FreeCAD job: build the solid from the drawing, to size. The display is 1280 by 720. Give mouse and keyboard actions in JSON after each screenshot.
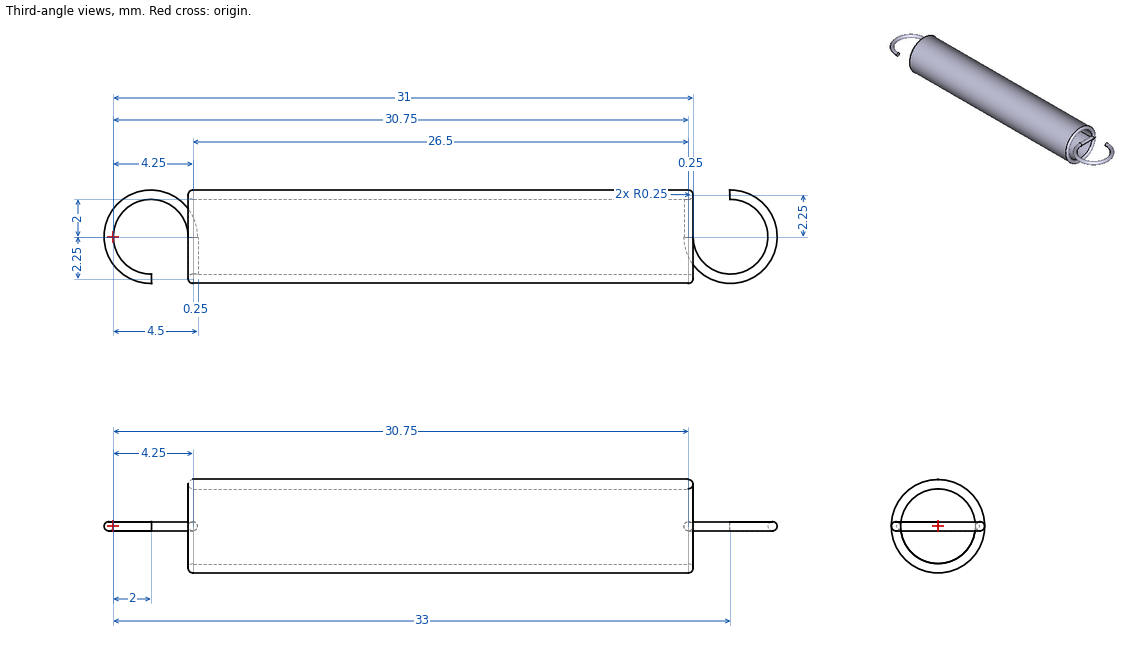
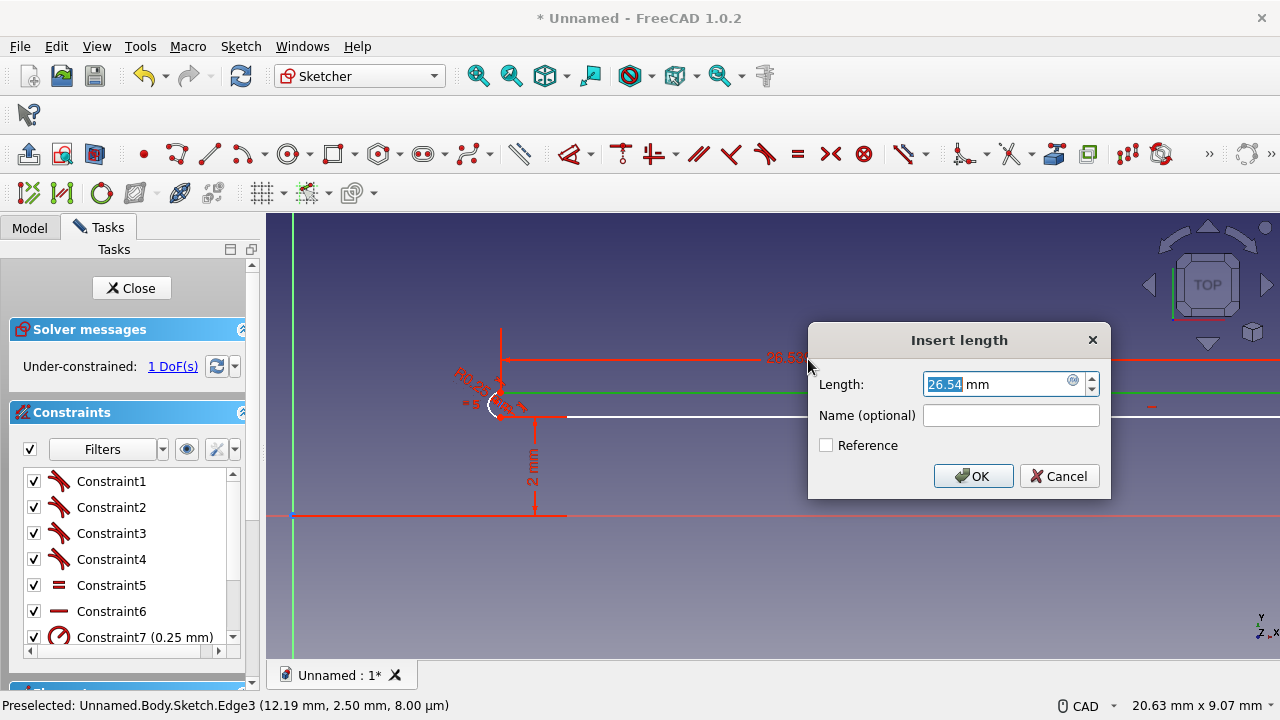
{"action": "type", "text": "26.5"}
{"action": "key", "text": "Return"}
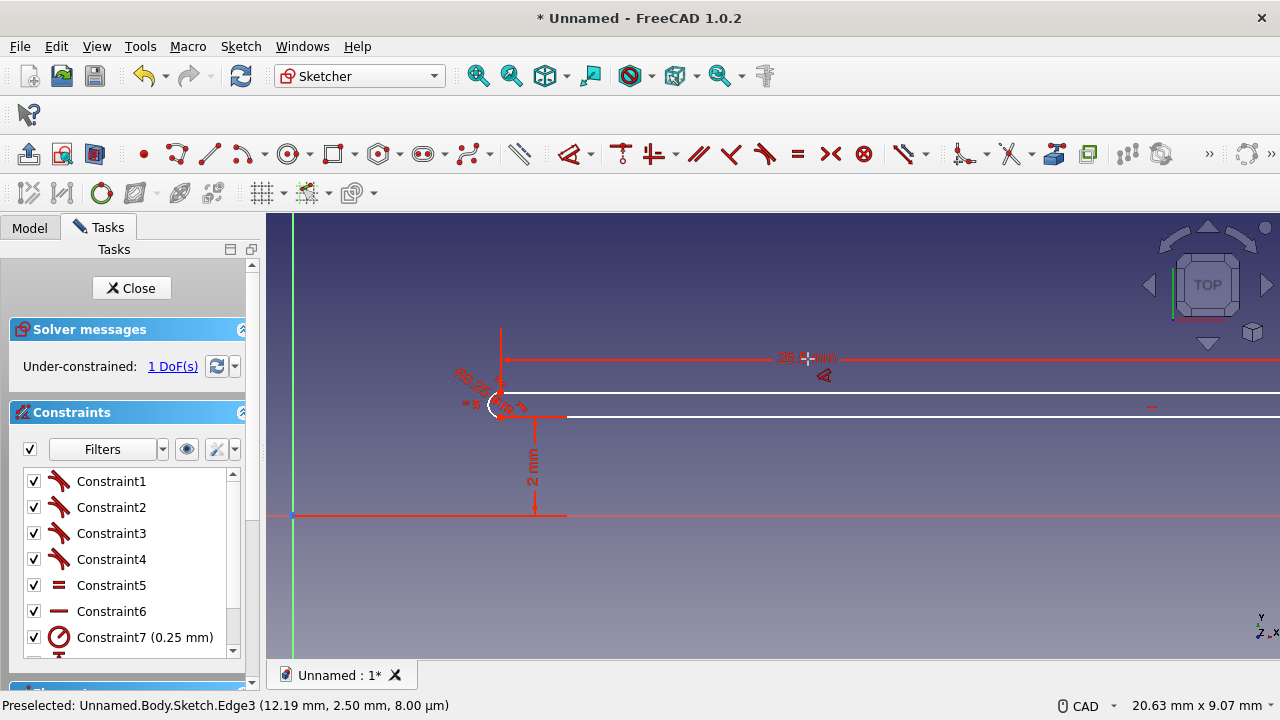
{"action": "left_click", "coordinate": [501, 393]}
{"action": "left_click", "coordinate": [397, 550]}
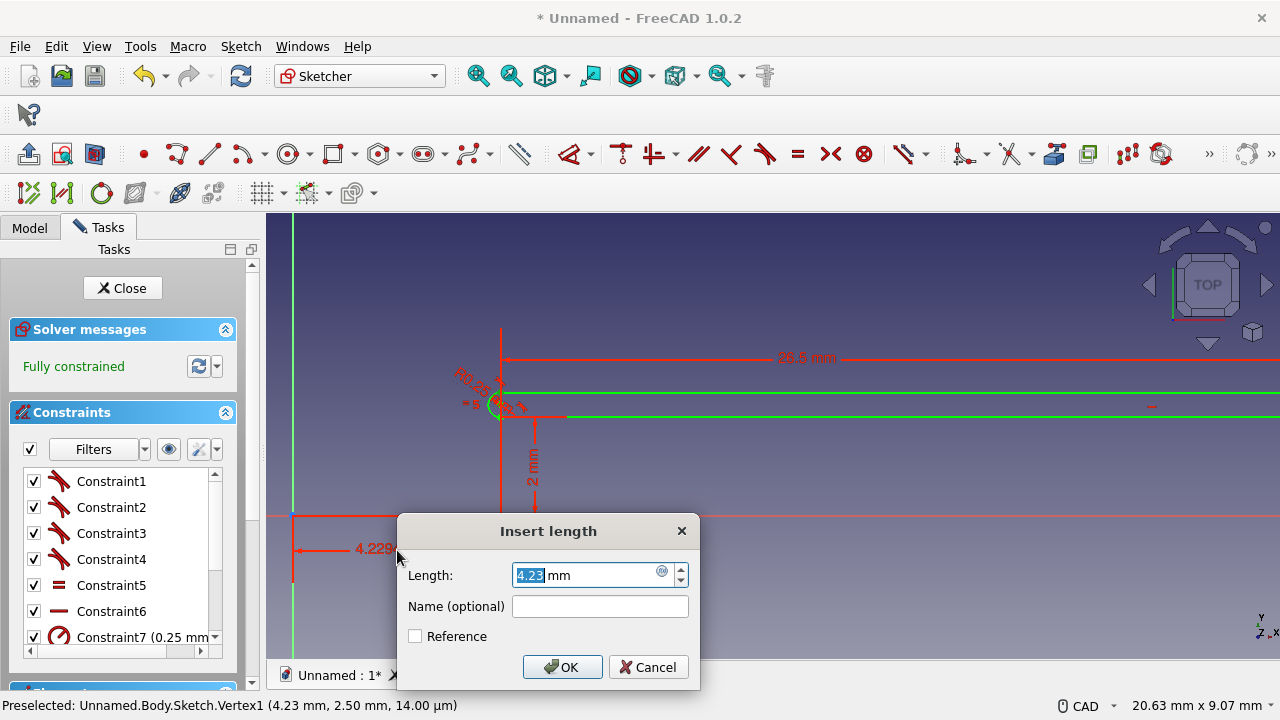
{"action": "type", "text": "4.25"}
{"action": "key", "text": "Return"}
{"action": "key", "text": "Escape"}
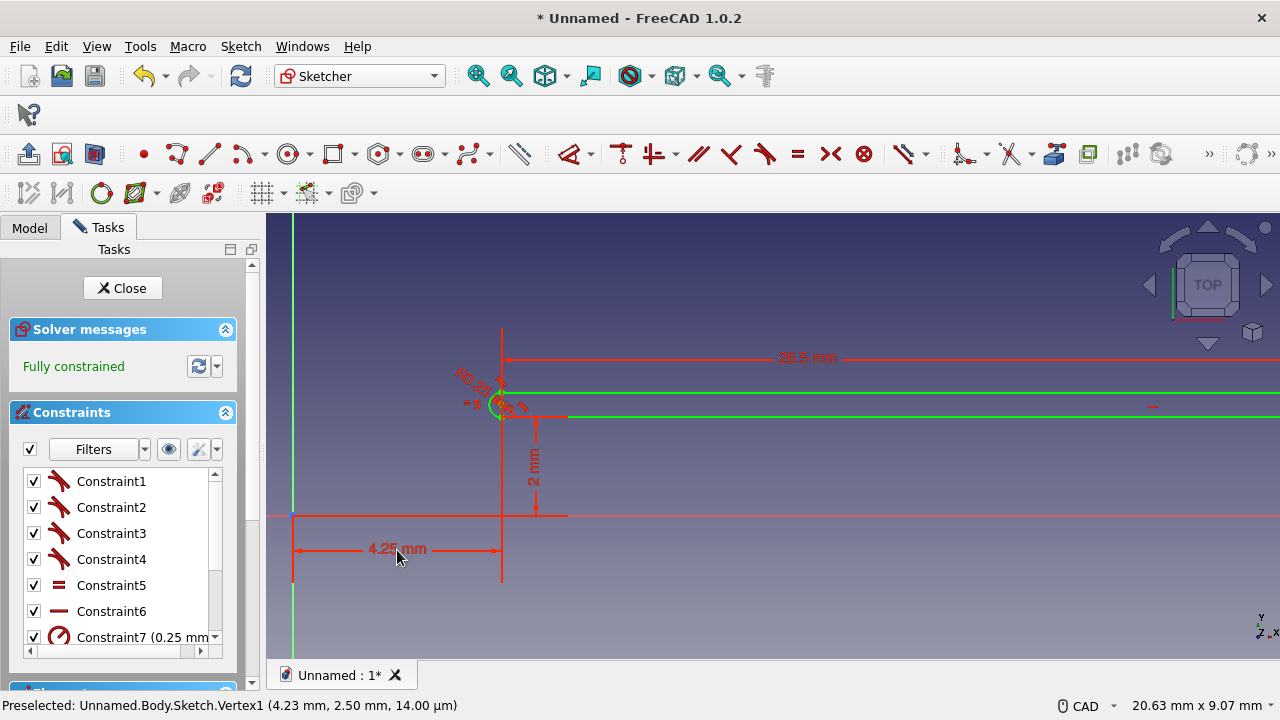
{"action": "left_click", "coordinate": [123, 288]}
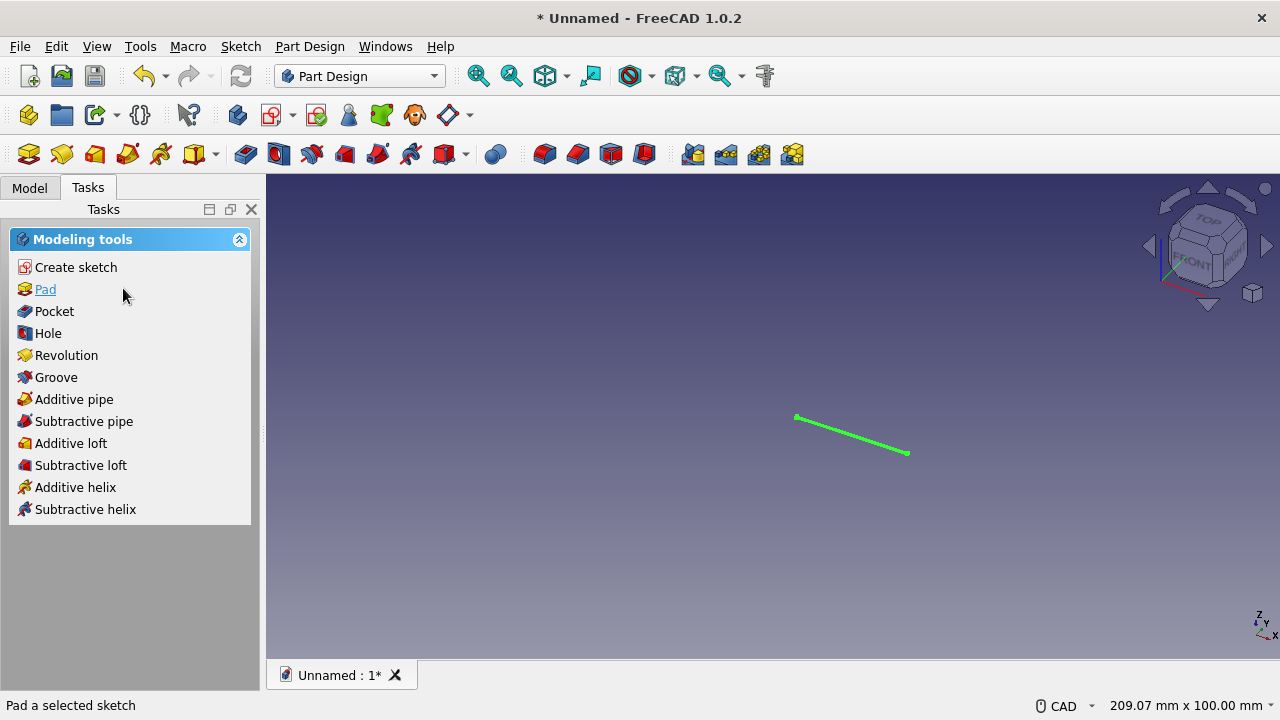
{"action": "left_click", "coordinate": [62, 154]}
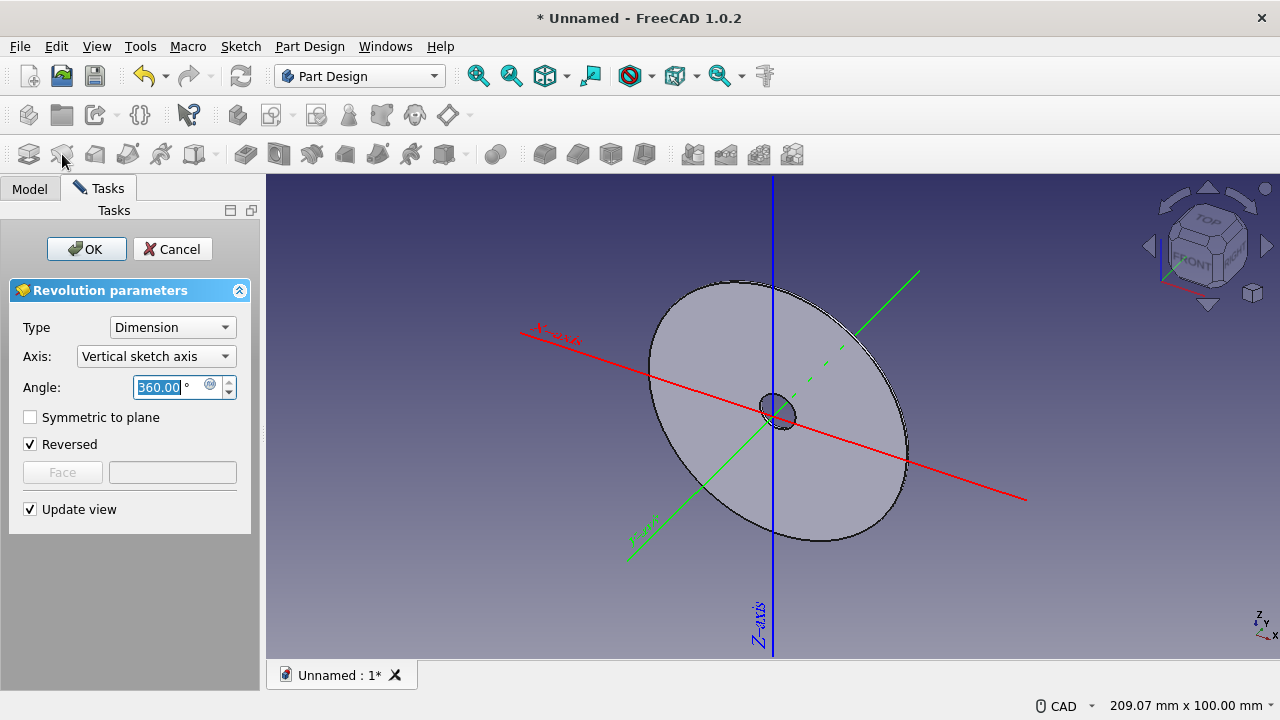
{"action": "left_click", "coordinate": [157, 356]}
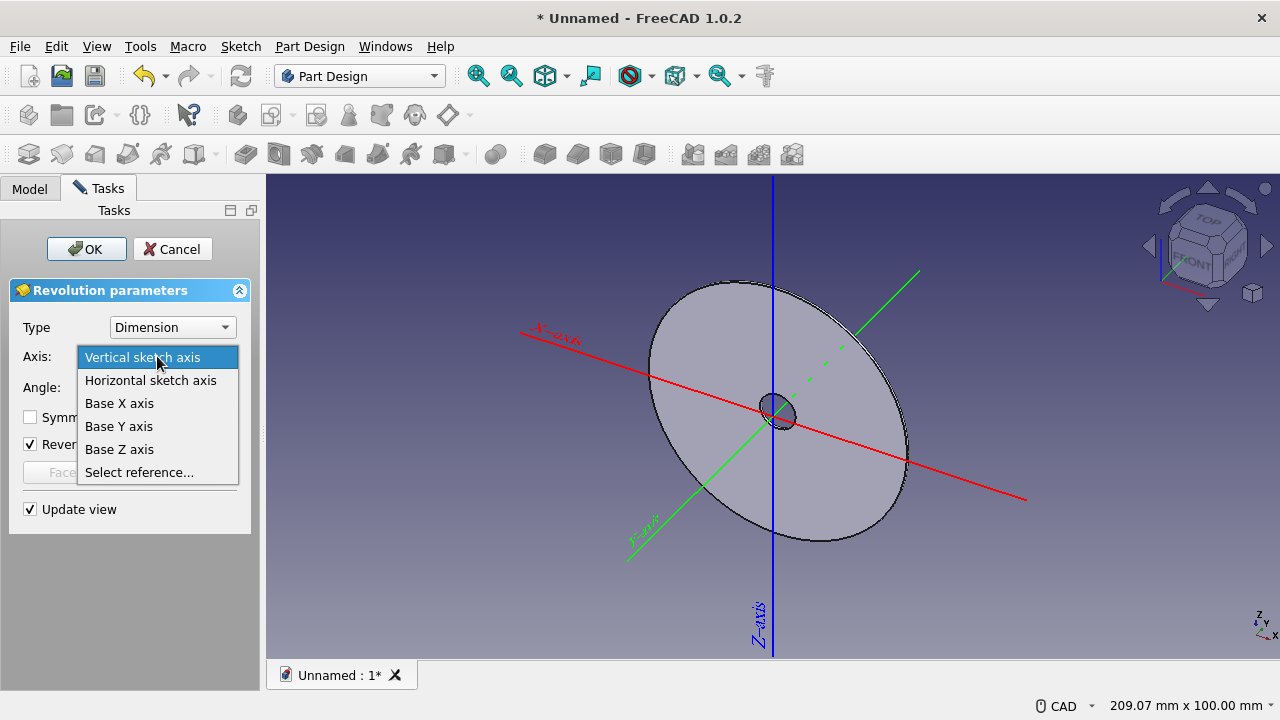
{"action": "left_click", "coordinate": [156, 380]}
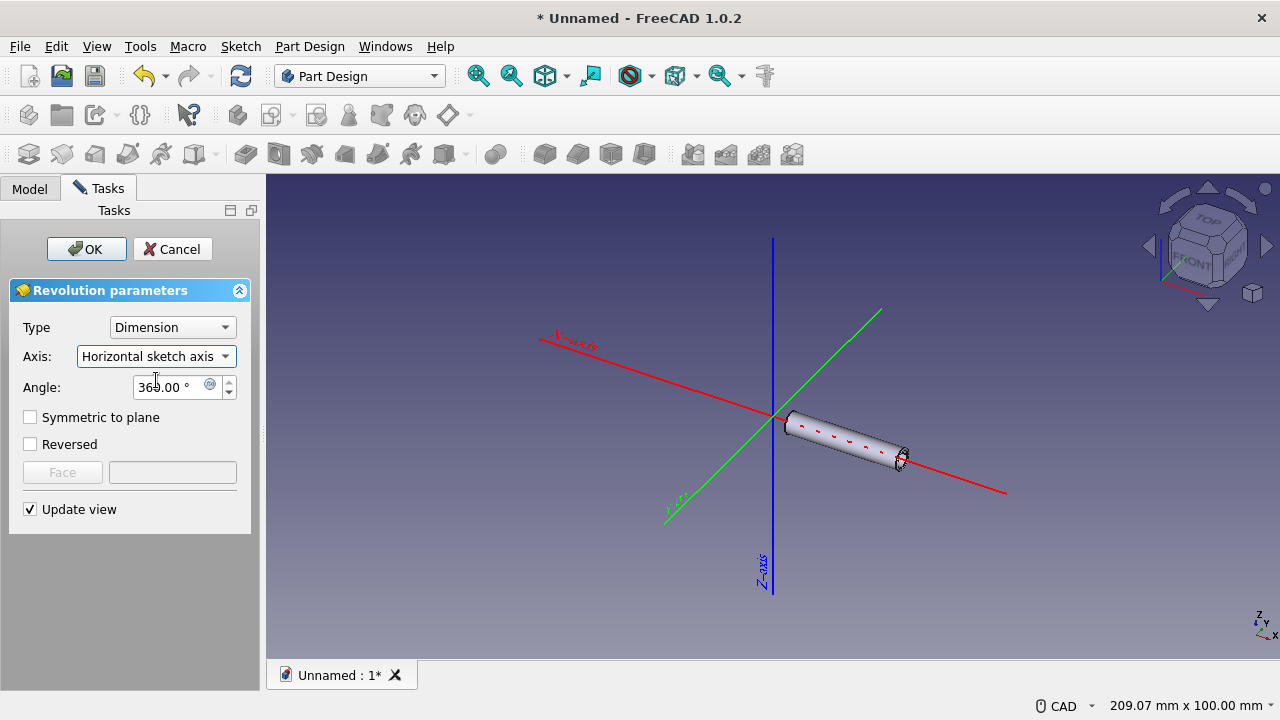
{"action": "left_click", "coordinate": [87, 249]}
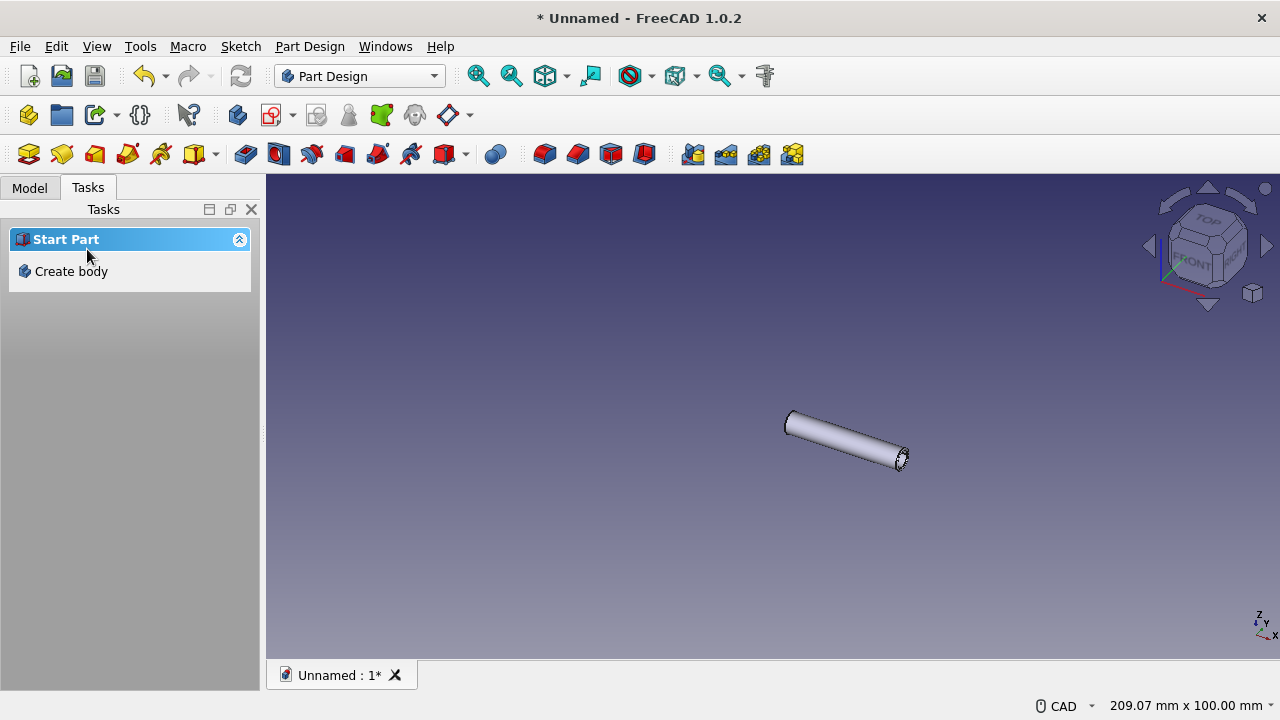
{"action": "key", "text": "v f"}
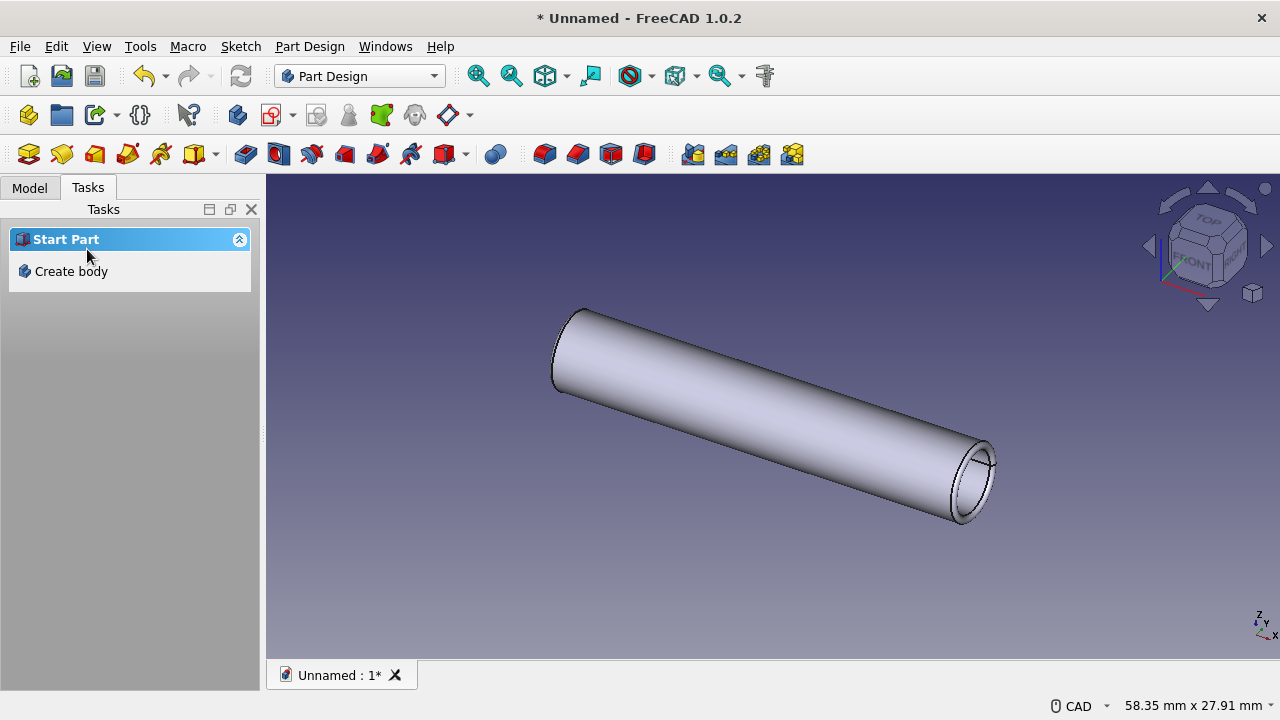
{"action": "left_click", "coordinate": [270, 116]}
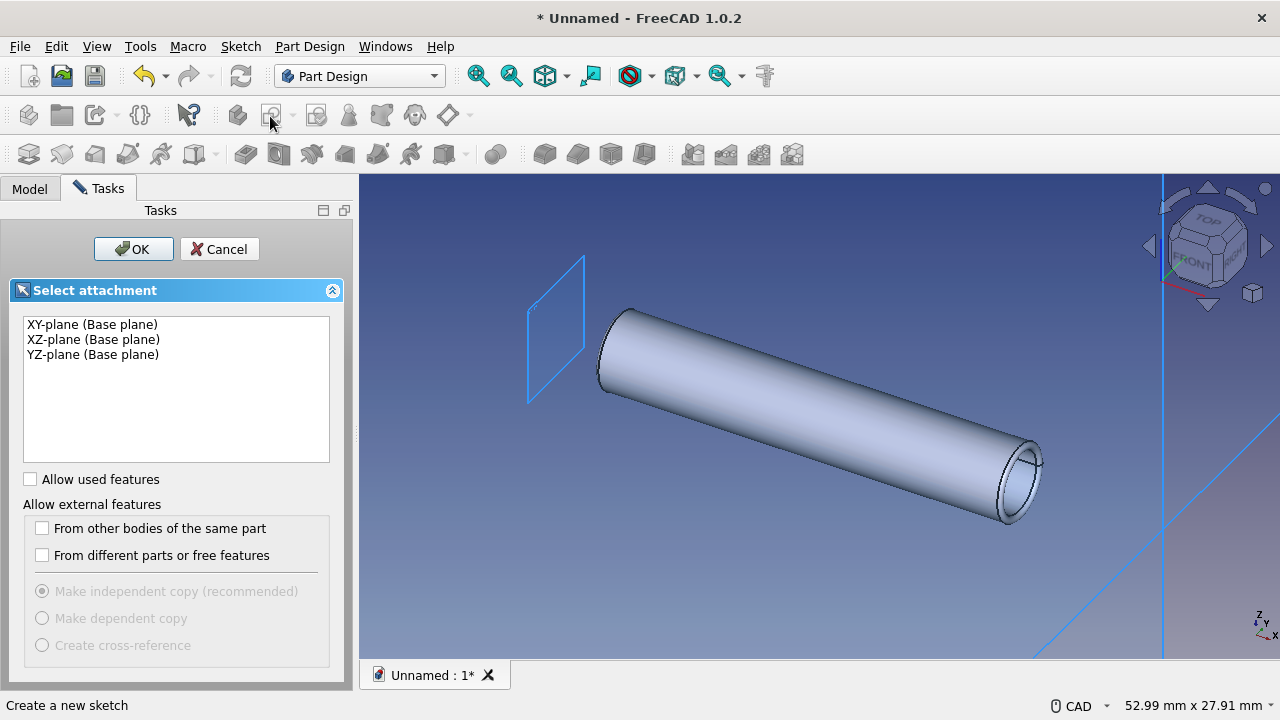
{"action": "left_click", "coordinate": [84, 324]}